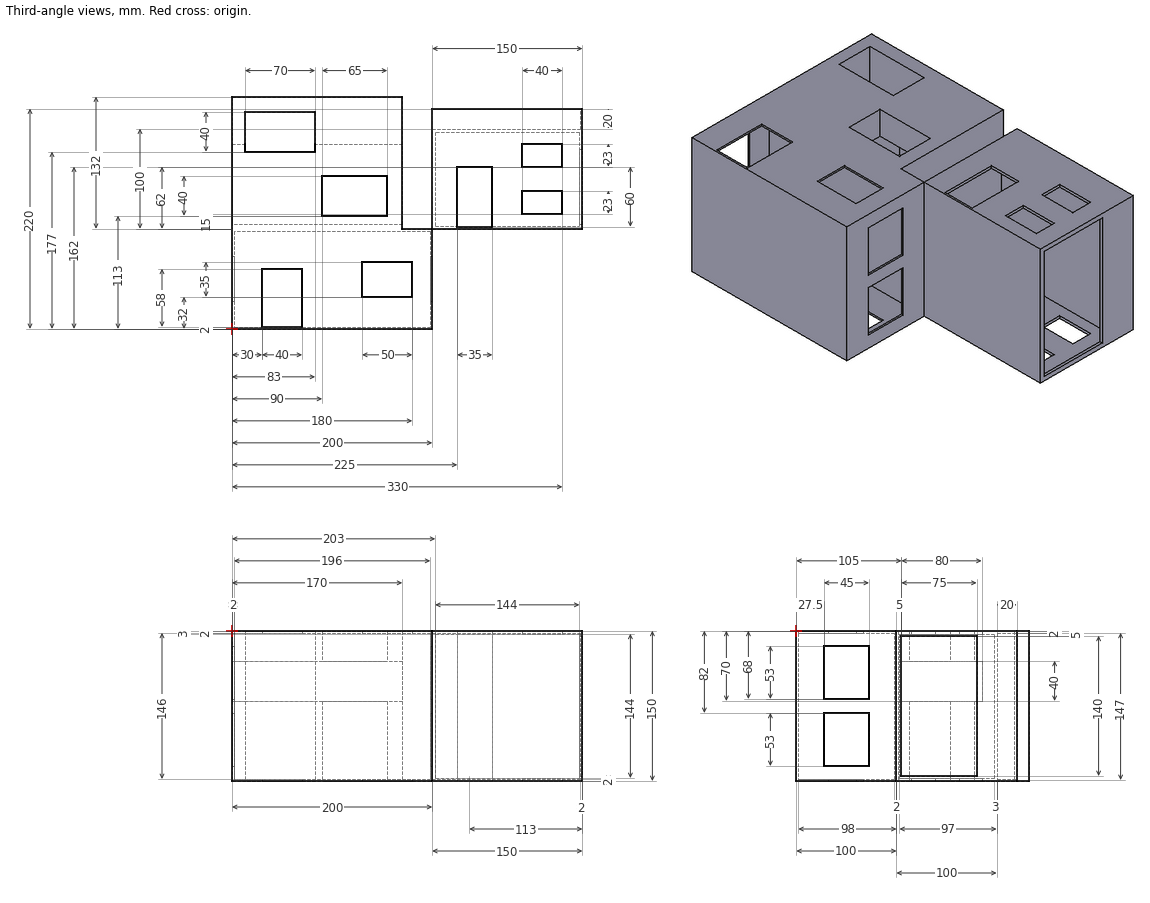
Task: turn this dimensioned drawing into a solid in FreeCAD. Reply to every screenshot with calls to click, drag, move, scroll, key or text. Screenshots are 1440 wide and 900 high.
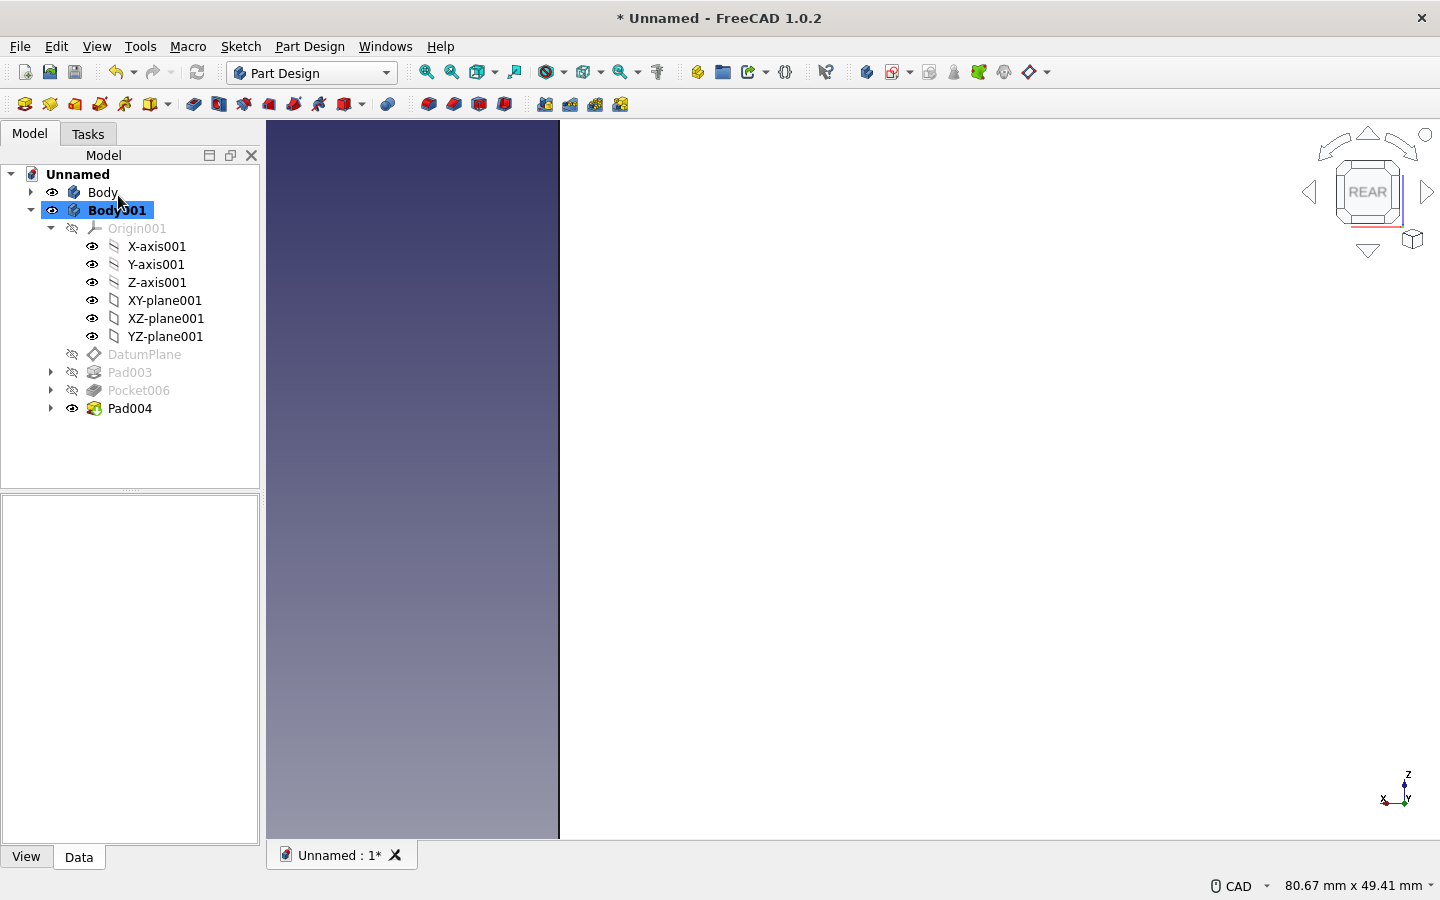
click(427, 72)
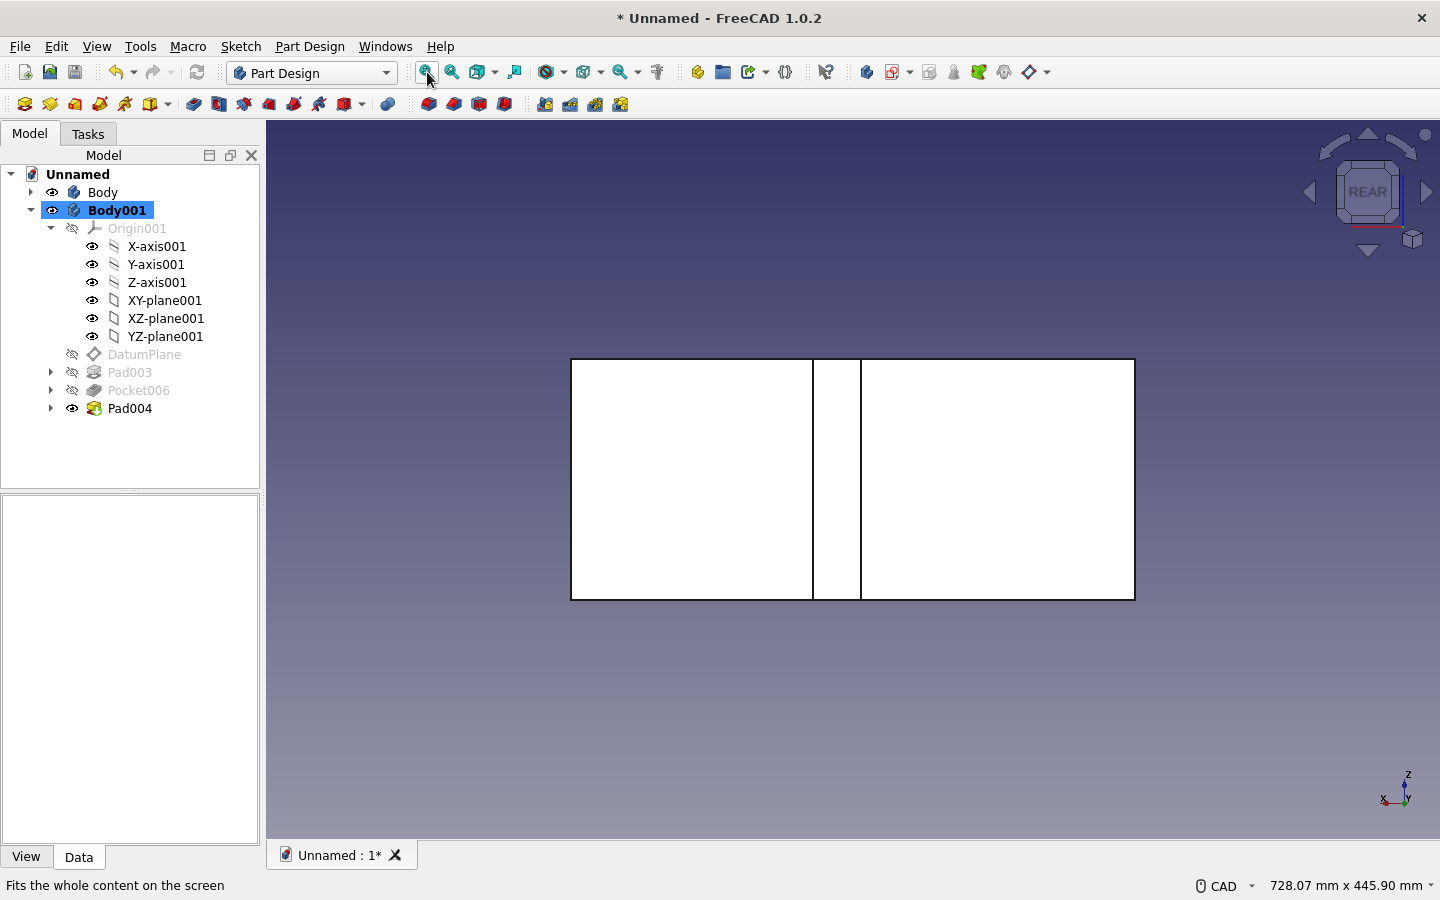
click(892, 72)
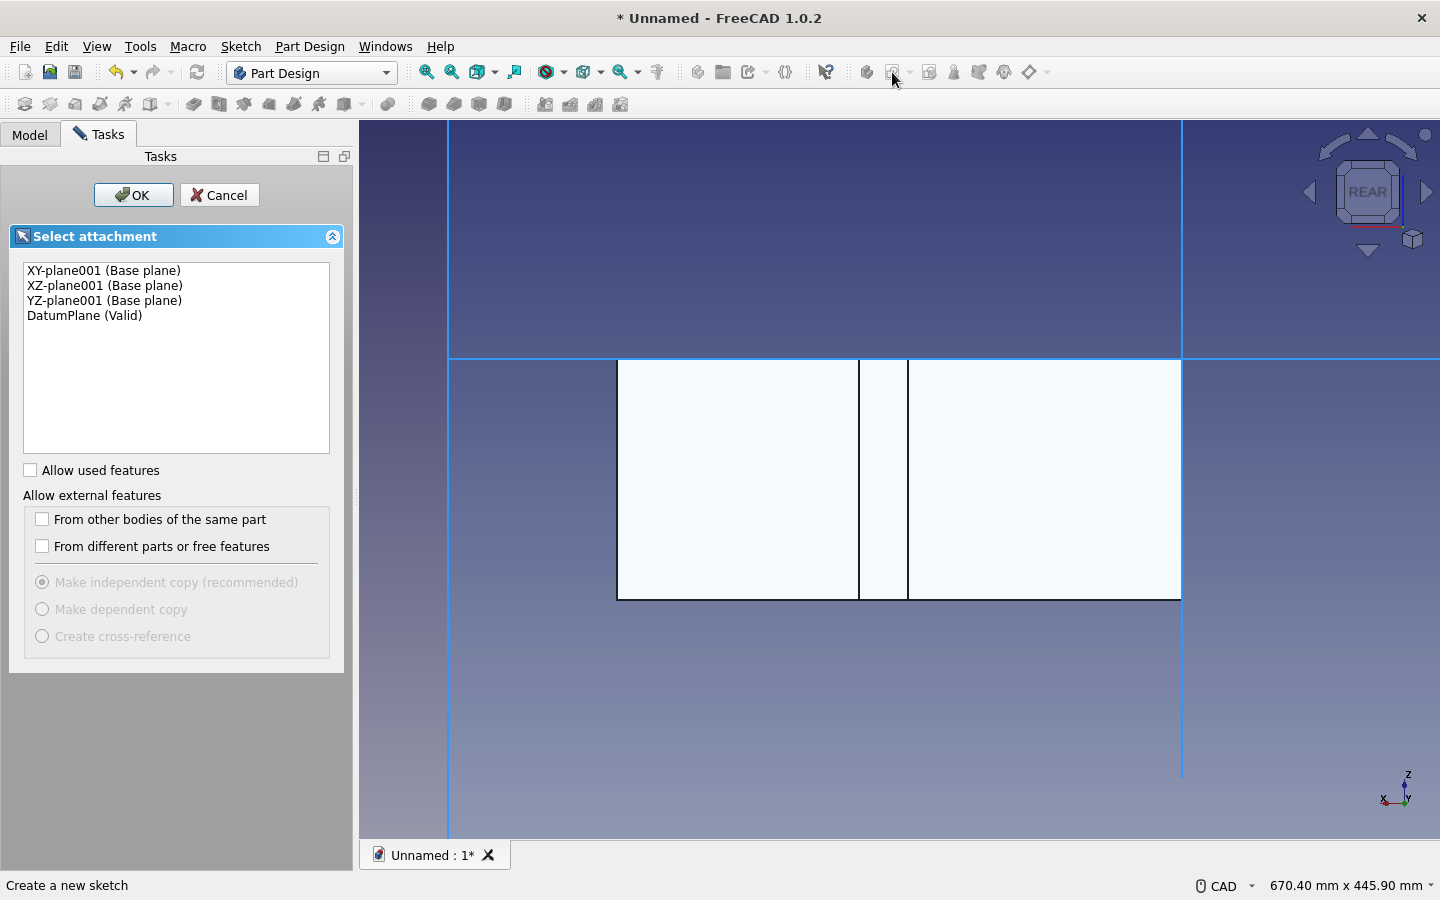
click(84, 270)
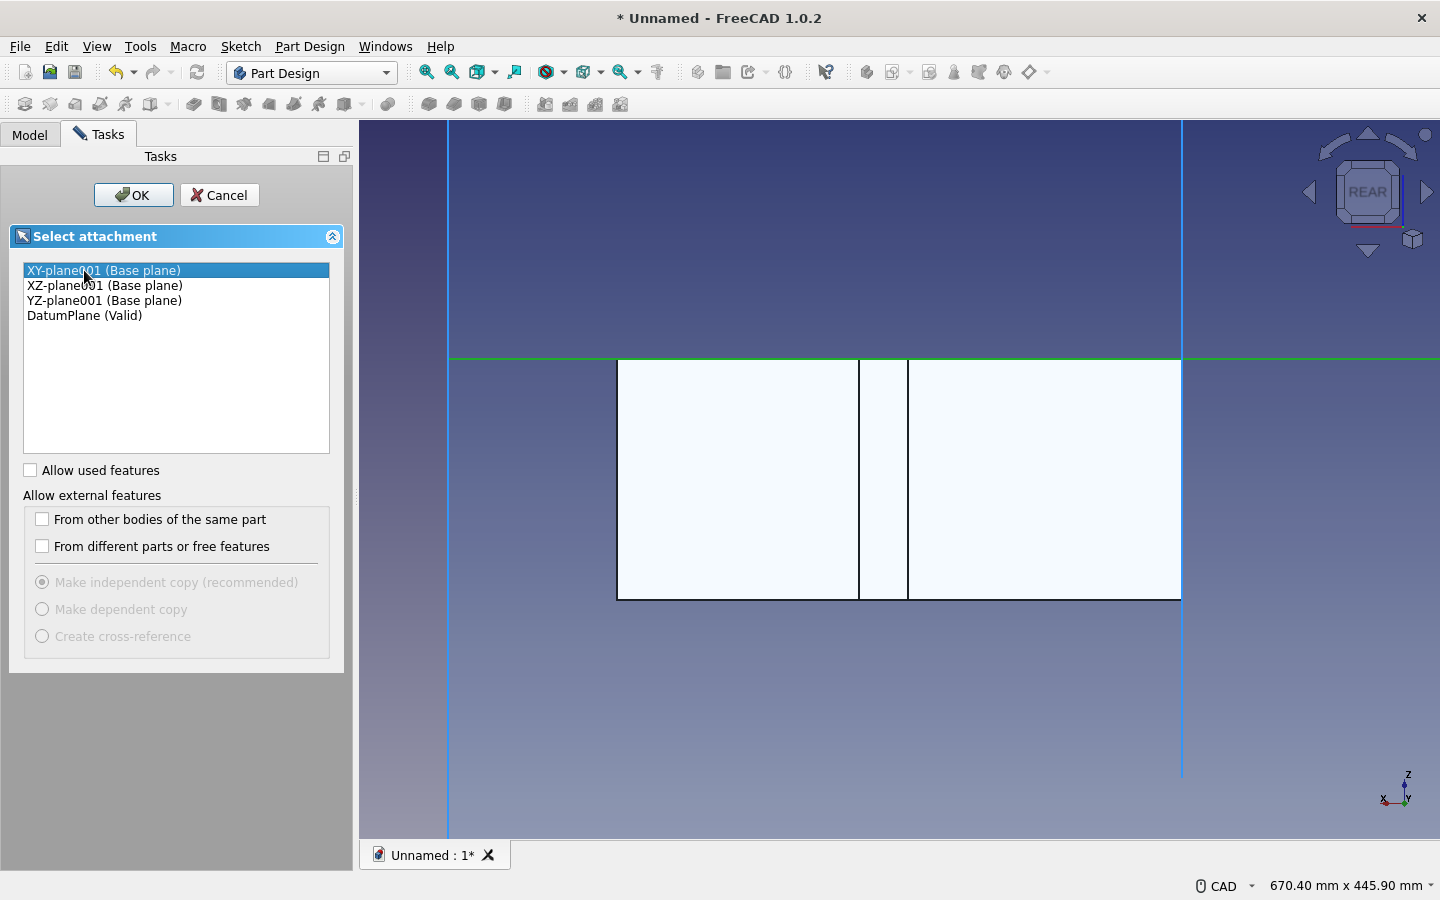
click(134, 195)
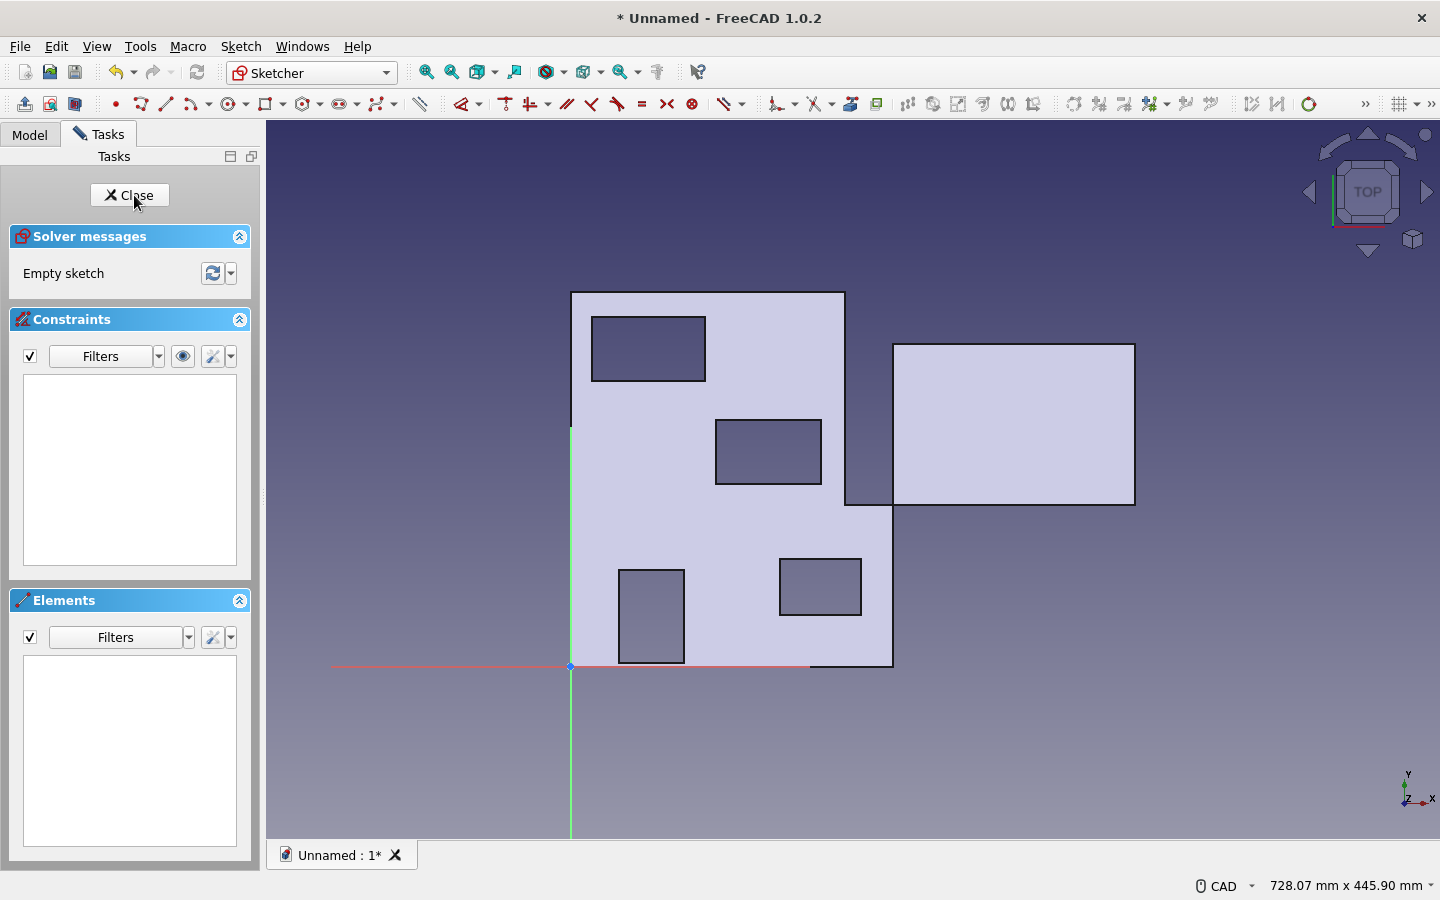
scroll(1007, 447, up, 8)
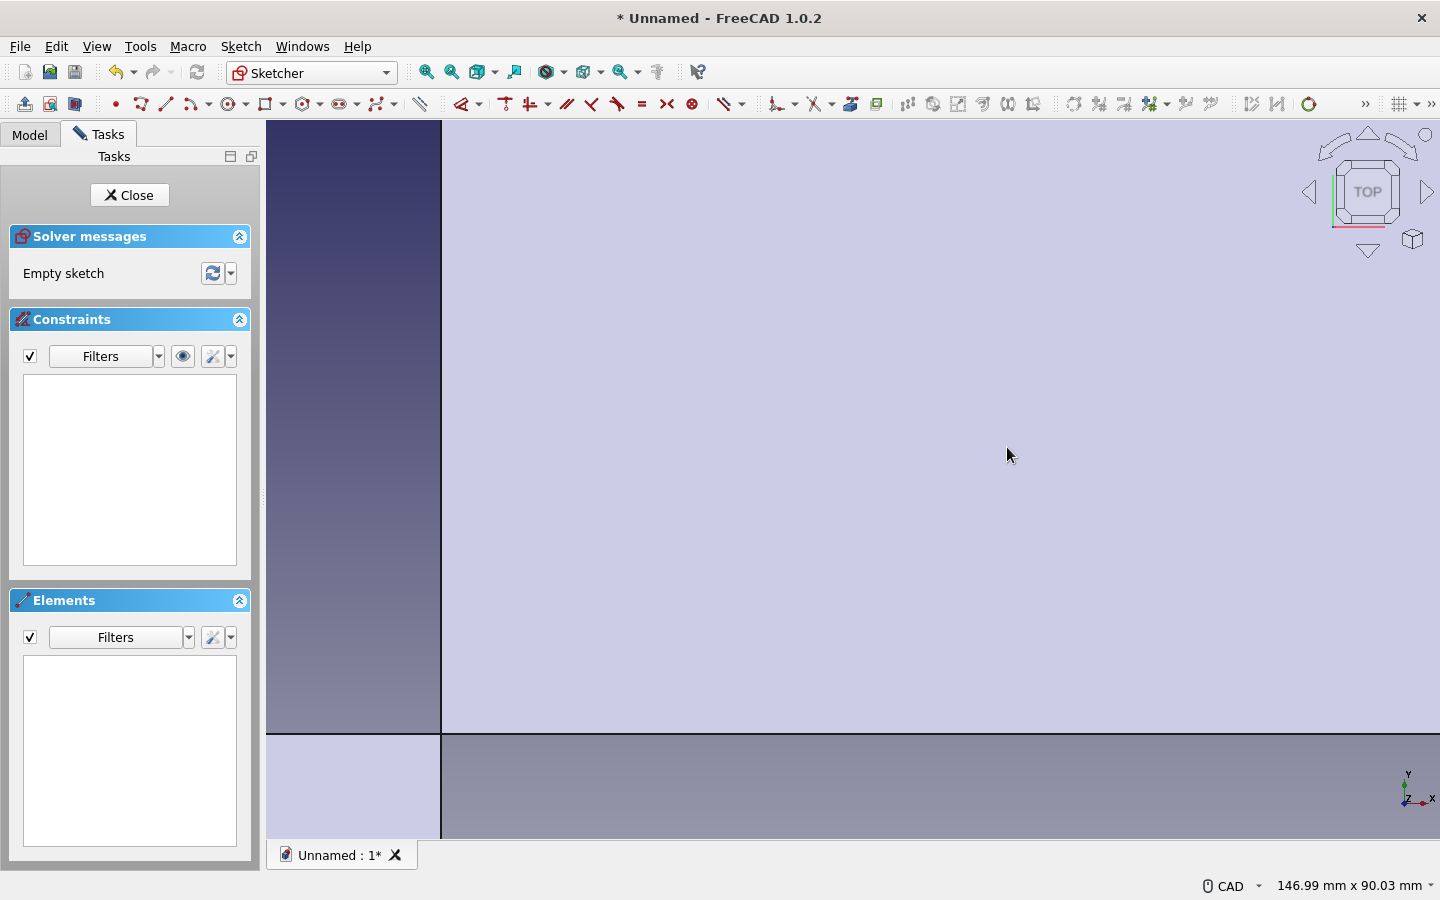
click(264, 104)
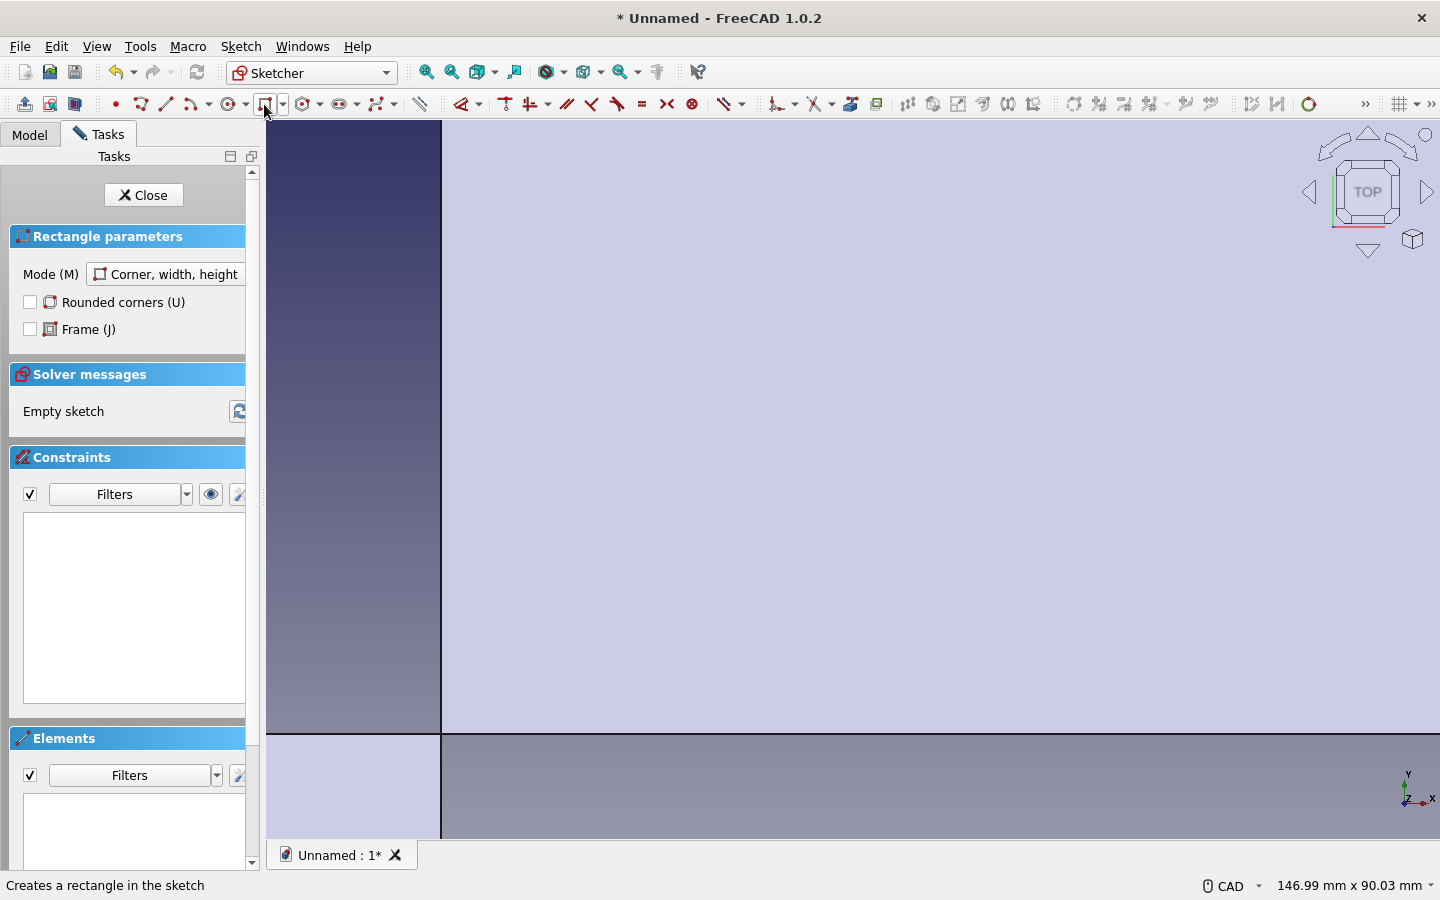
click(641, 239)
move(921, 718)